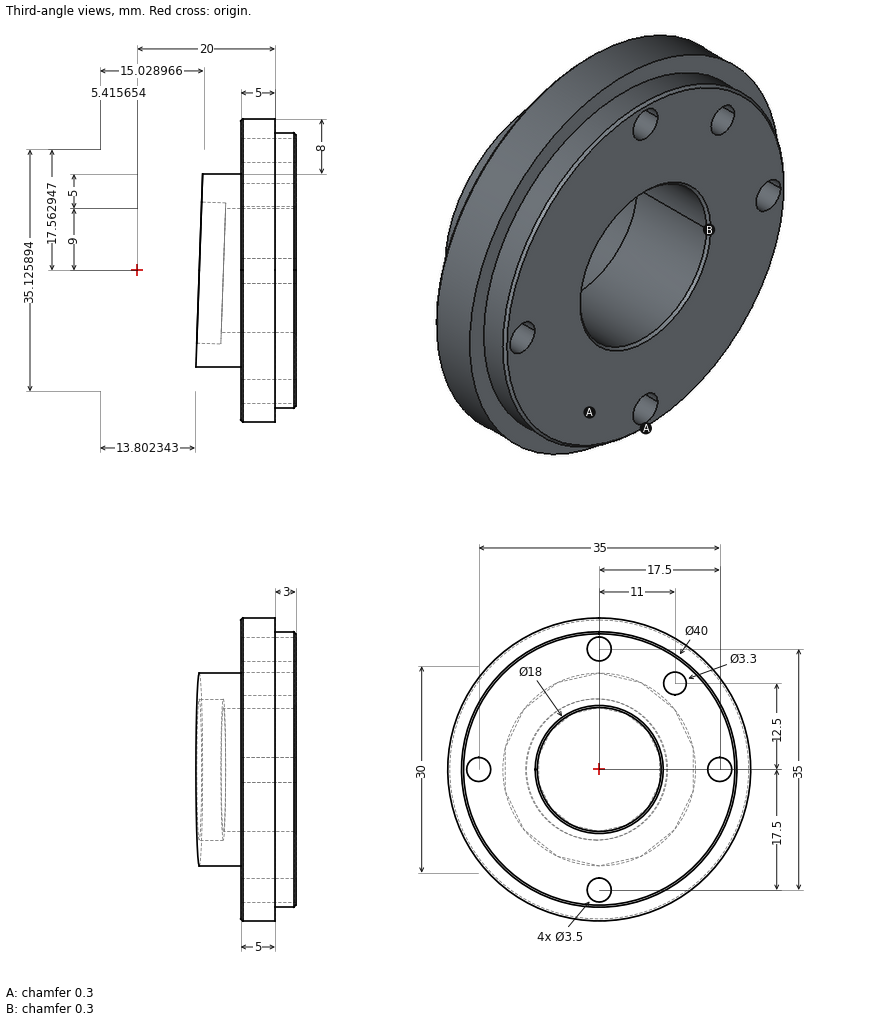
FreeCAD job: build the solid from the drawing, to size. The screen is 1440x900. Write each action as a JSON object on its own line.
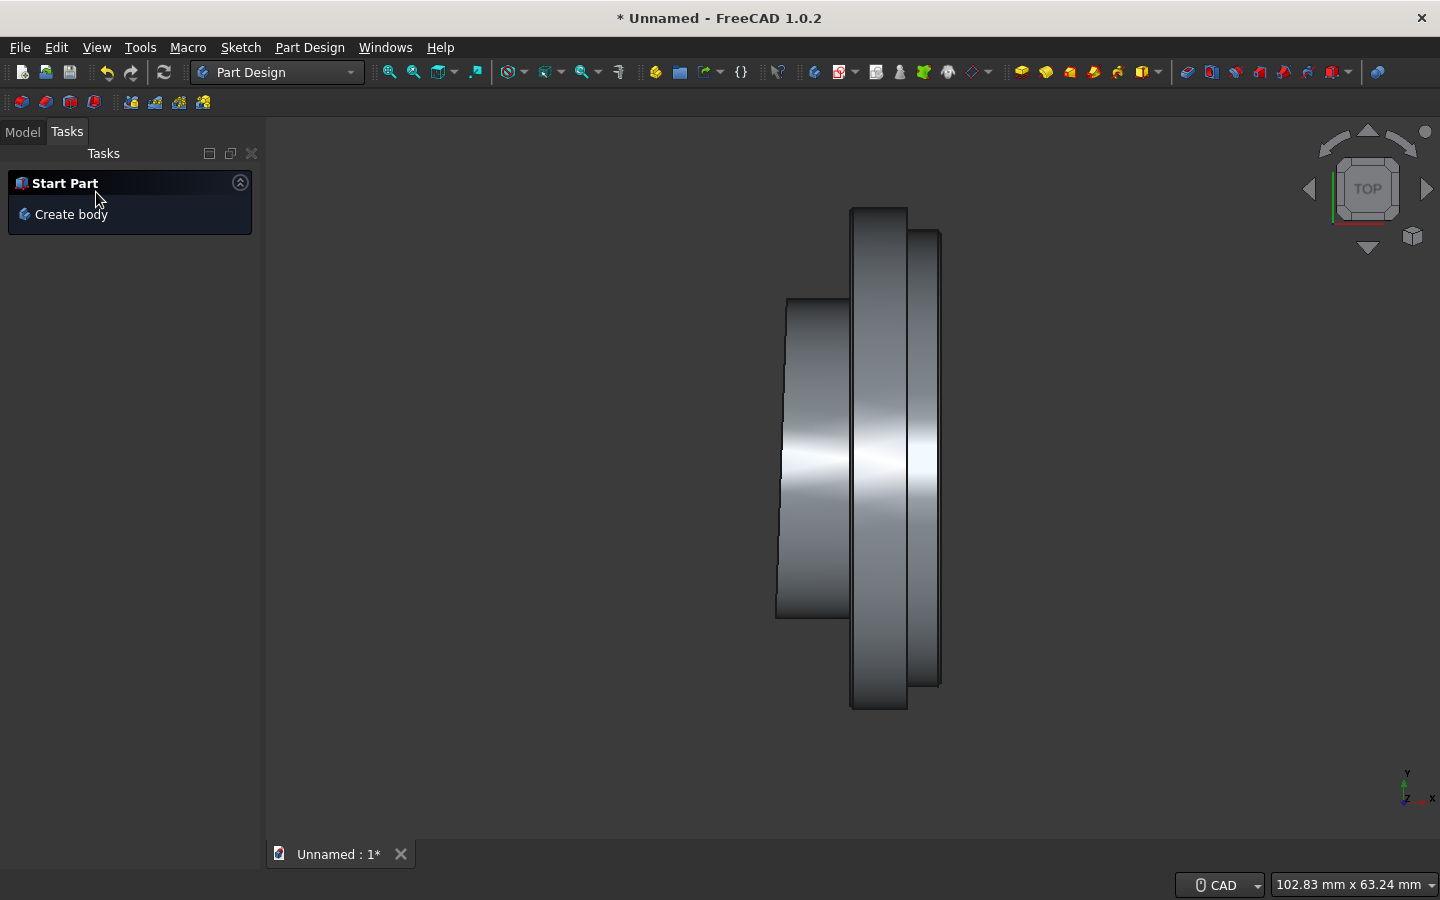
{"action": "key", "text": "0"}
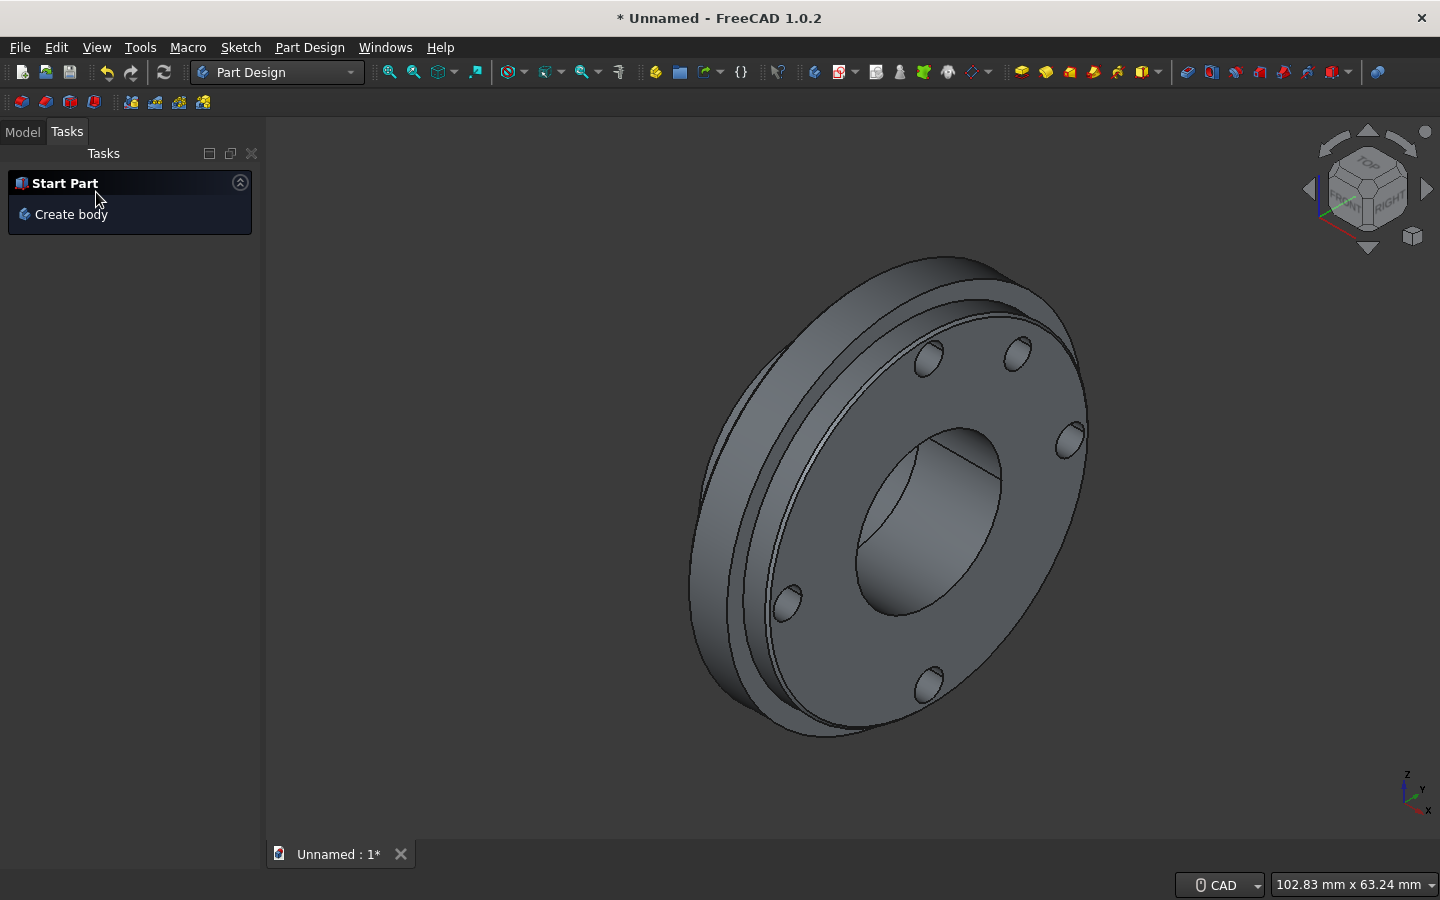
{"action": "left_click", "coordinate": [906, 614]}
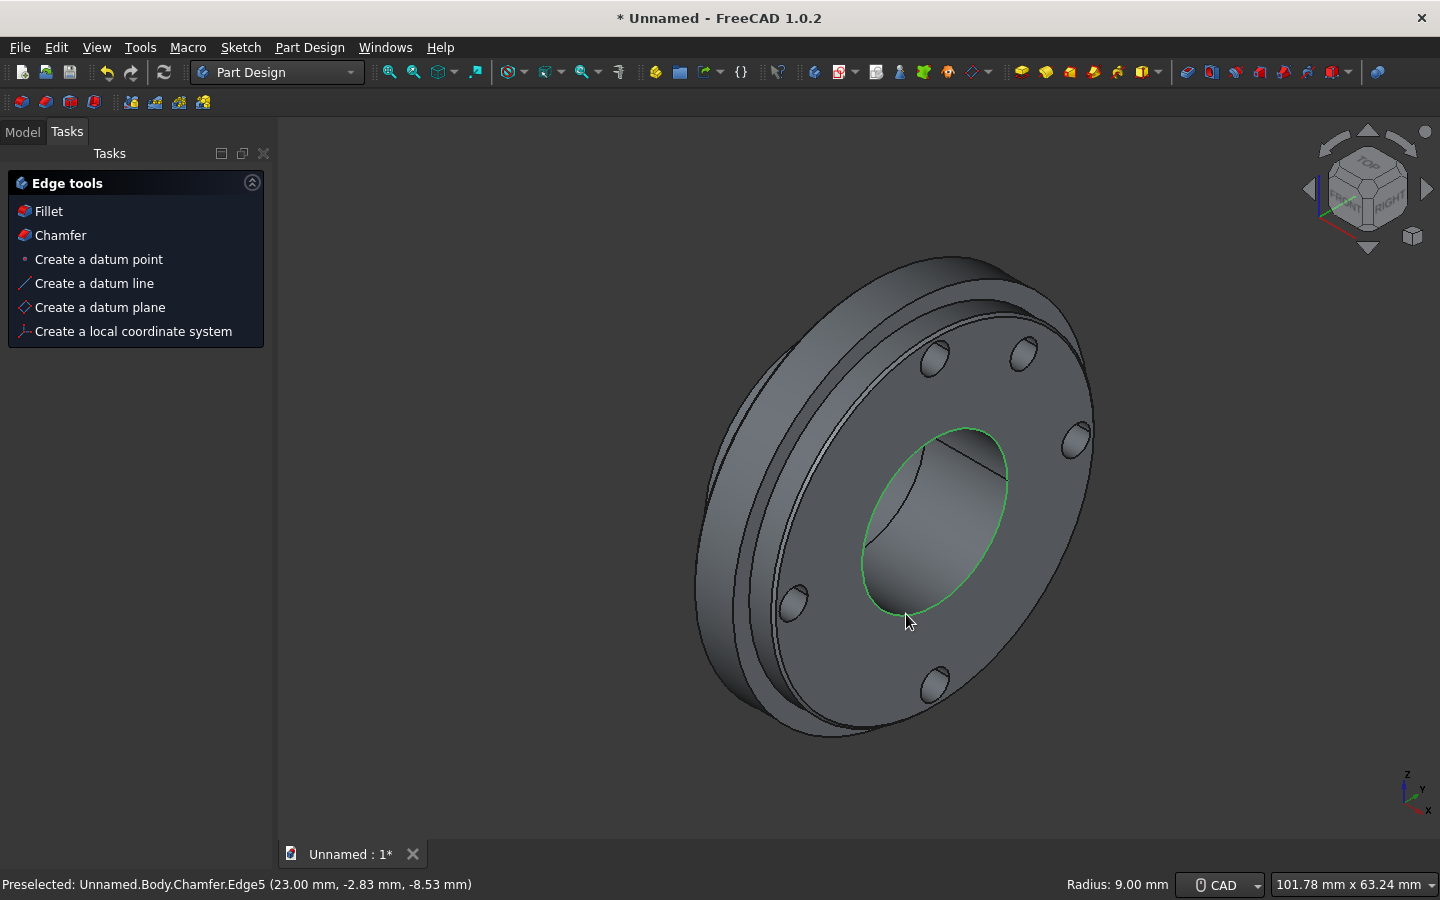
{"action": "left_click", "coordinate": [46, 102]}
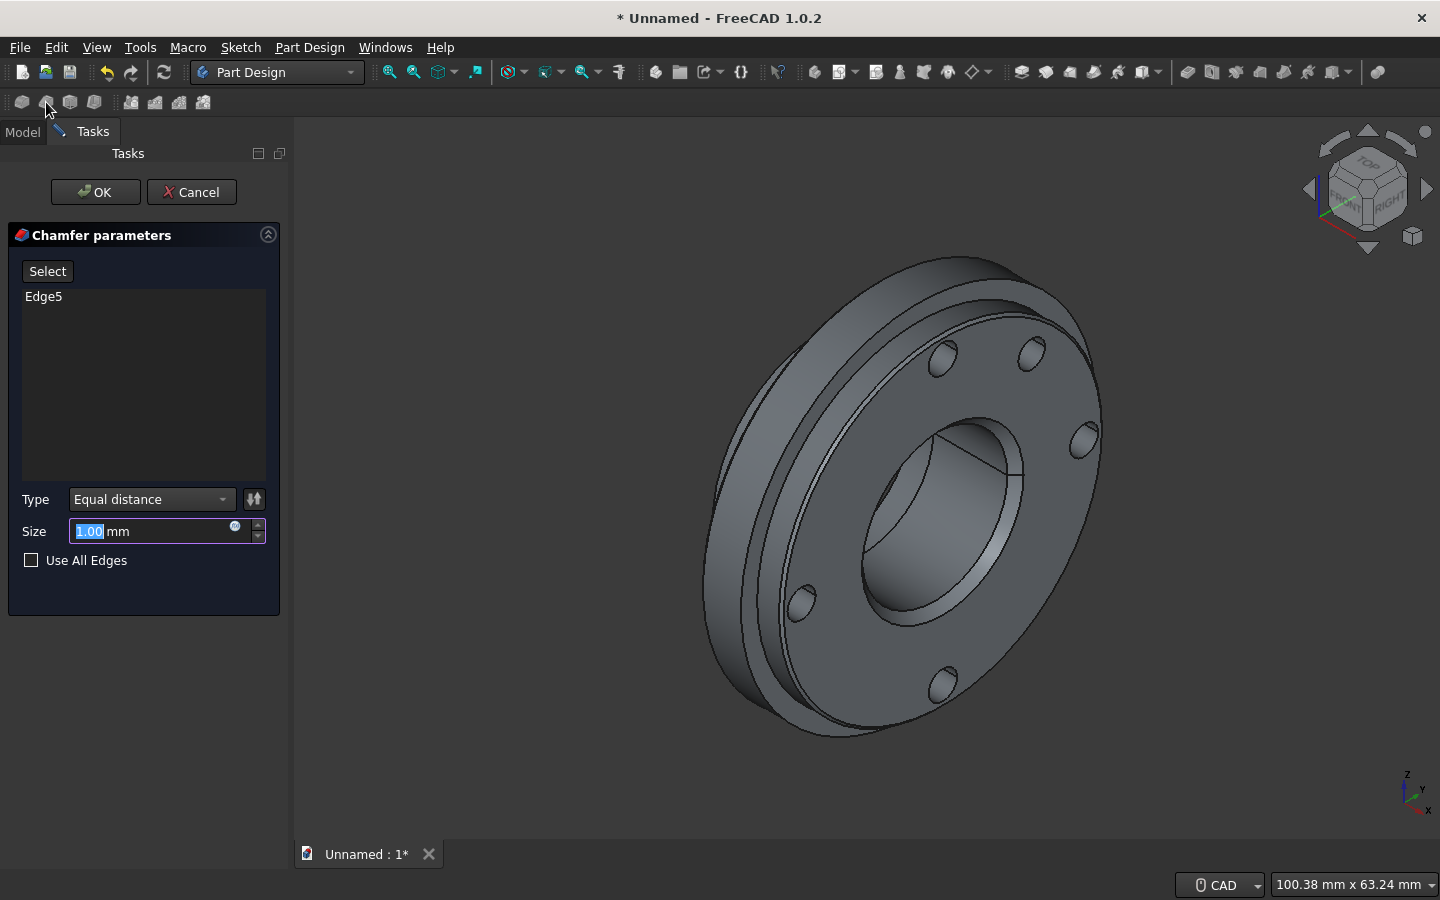
{"action": "type", "text": "0.3"}
{"action": "key", "text": "Tab"}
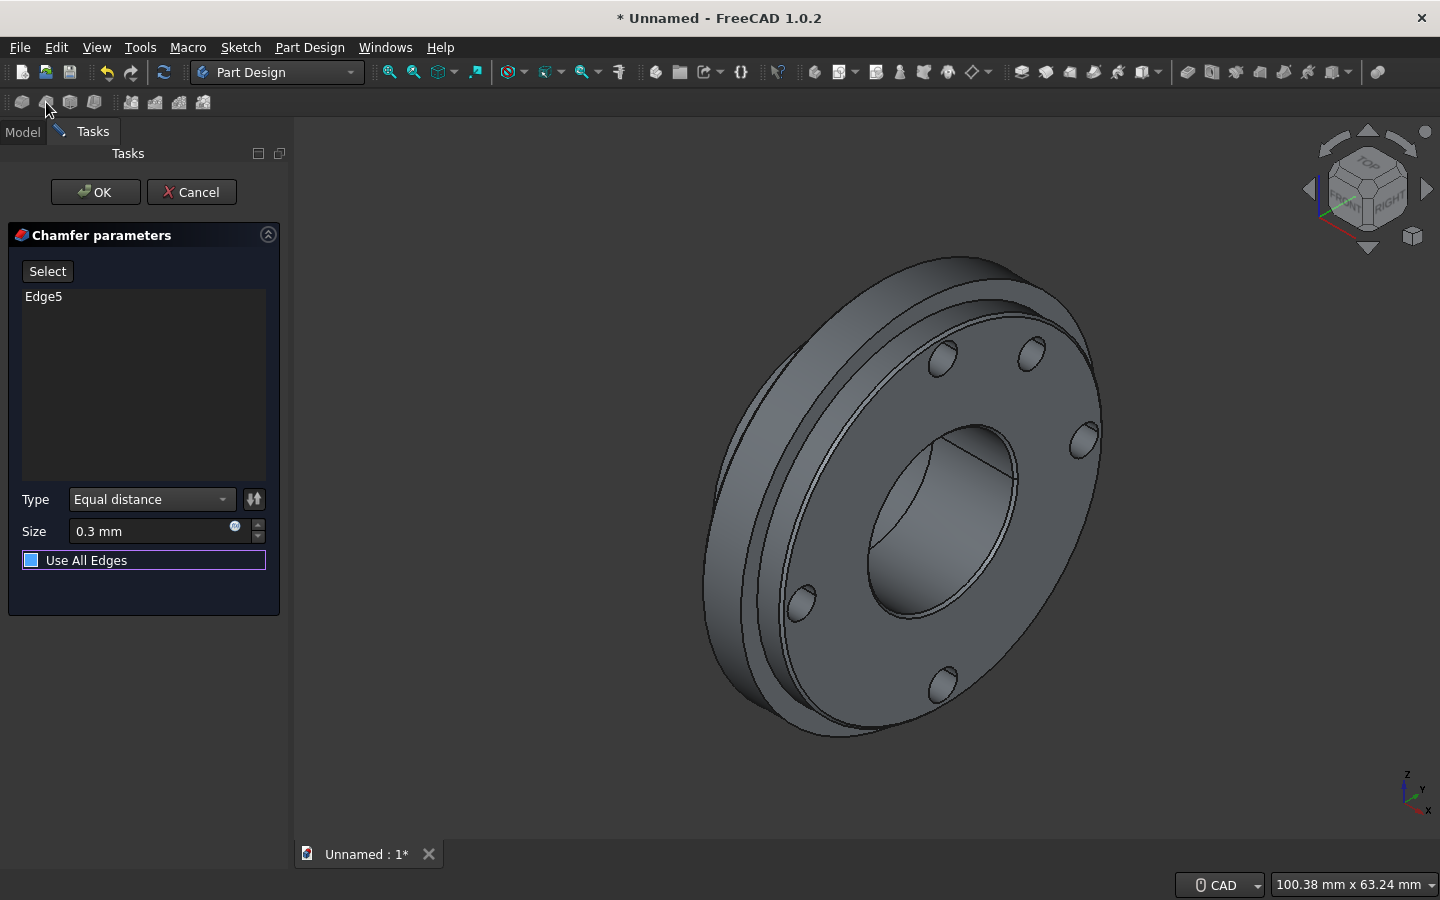
{"action": "left_click", "coordinate": [96, 192]}